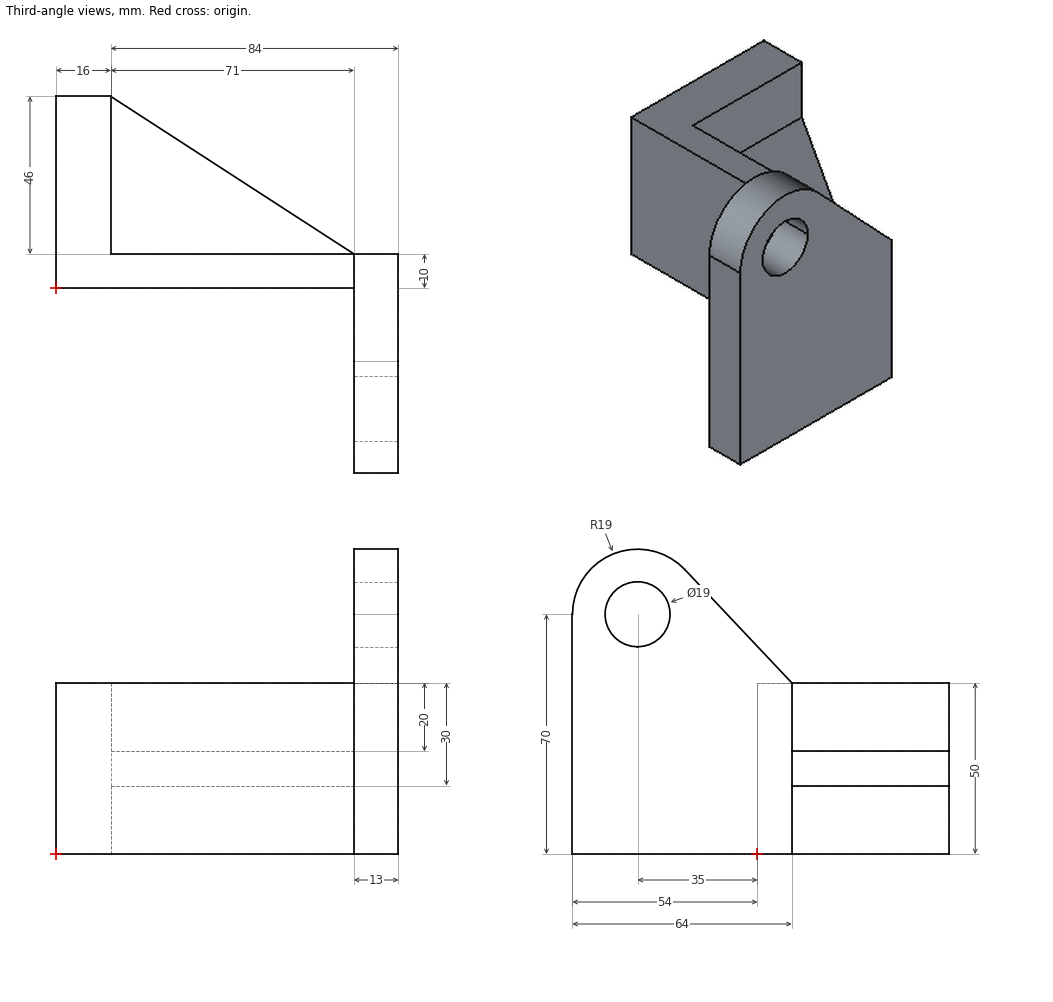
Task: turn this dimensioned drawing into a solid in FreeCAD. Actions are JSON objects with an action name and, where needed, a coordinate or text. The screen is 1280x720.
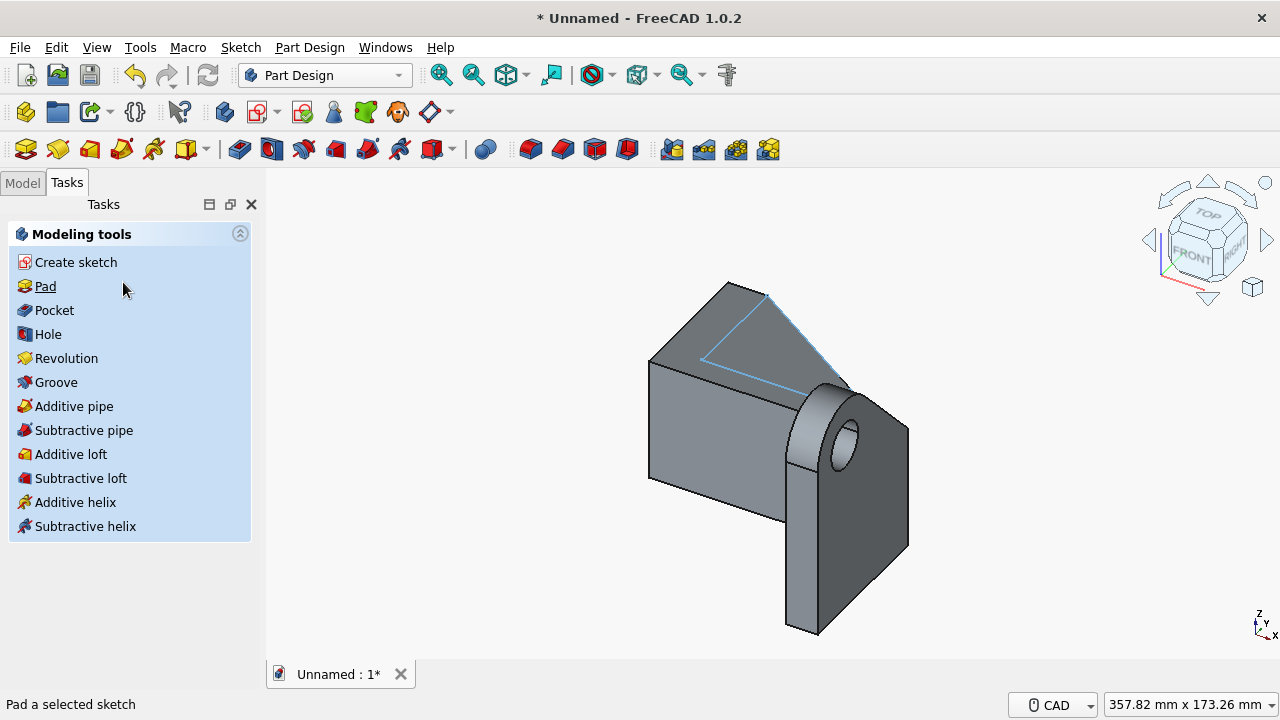
{"action": "left_click", "coordinate": [240, 150]}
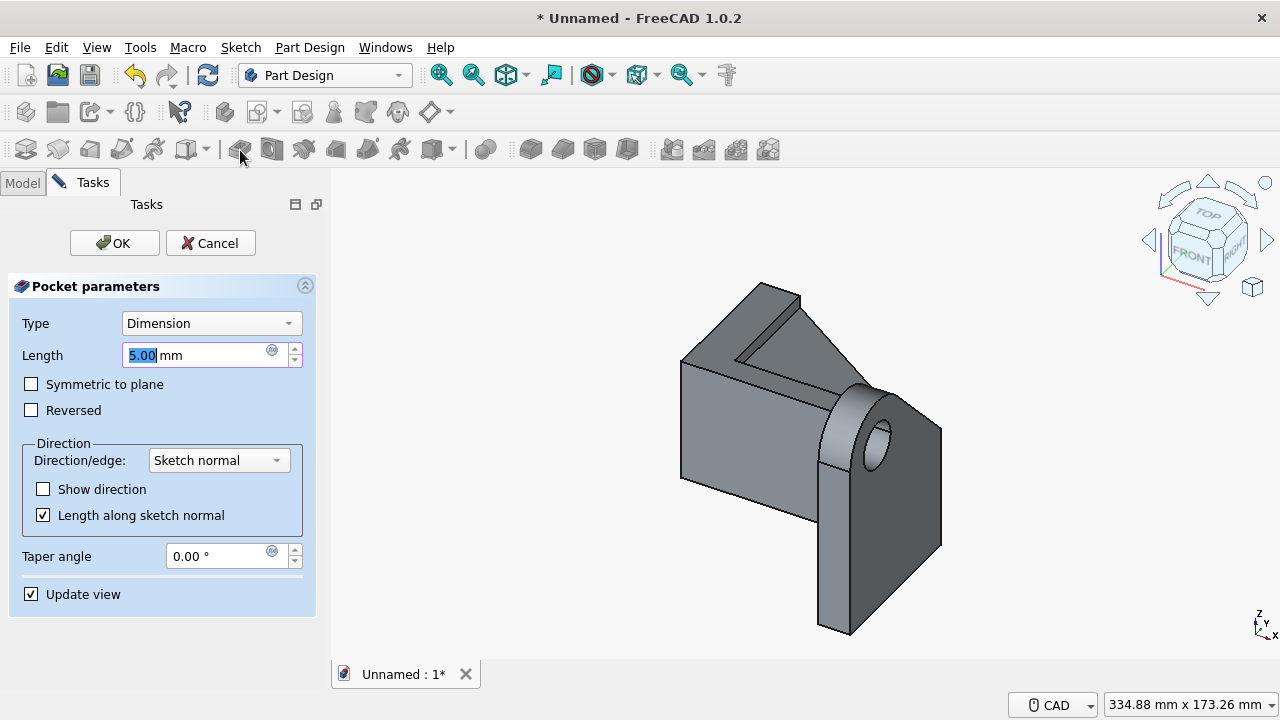
{"action": "type", "text": "20"}
{"action": "key", "text": "Tab"}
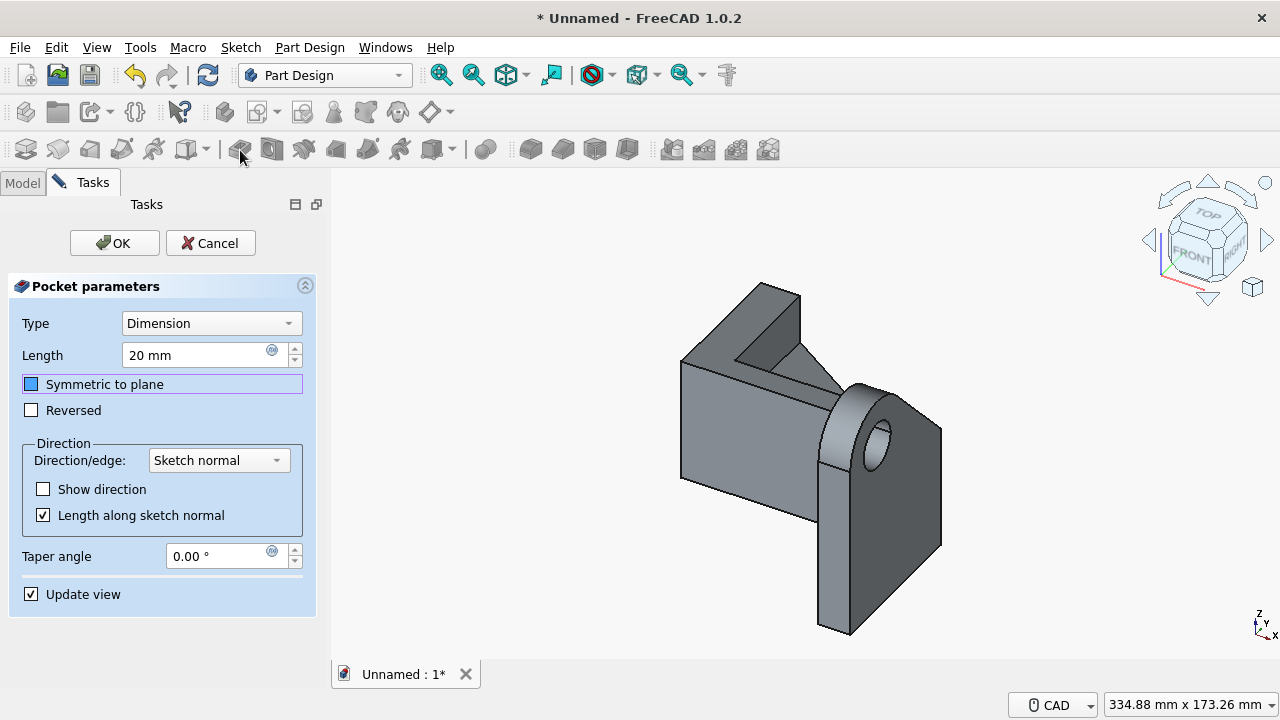
{"action": "left_click", "coordinate": [115, 243]}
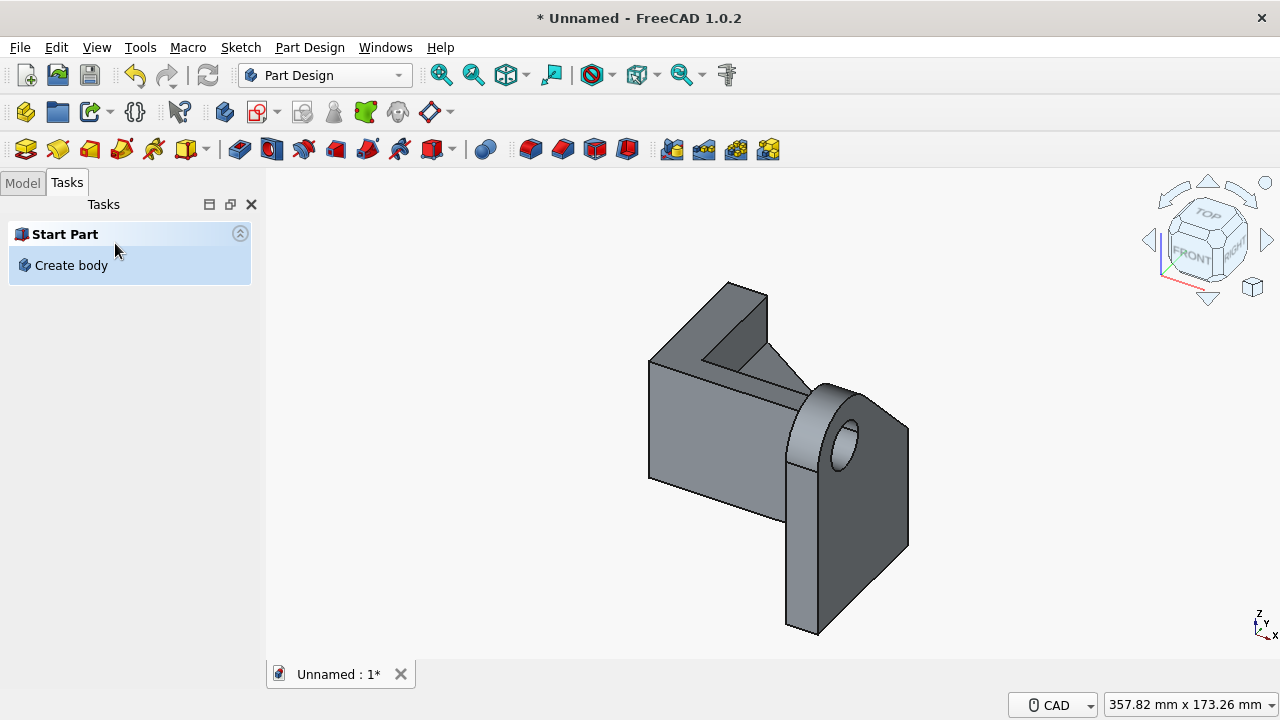
{"action": "key", "text": "0"}